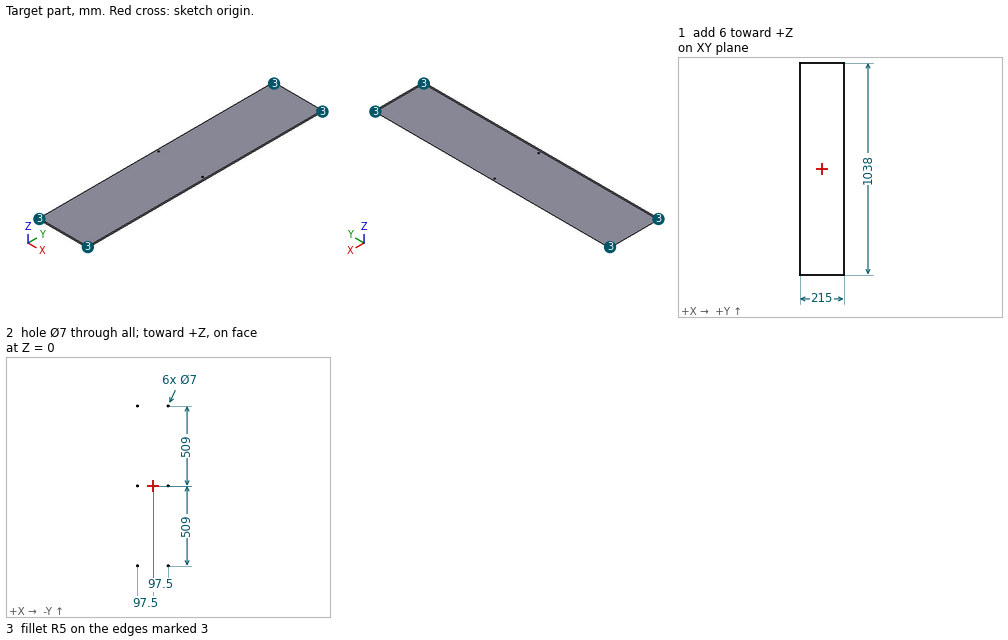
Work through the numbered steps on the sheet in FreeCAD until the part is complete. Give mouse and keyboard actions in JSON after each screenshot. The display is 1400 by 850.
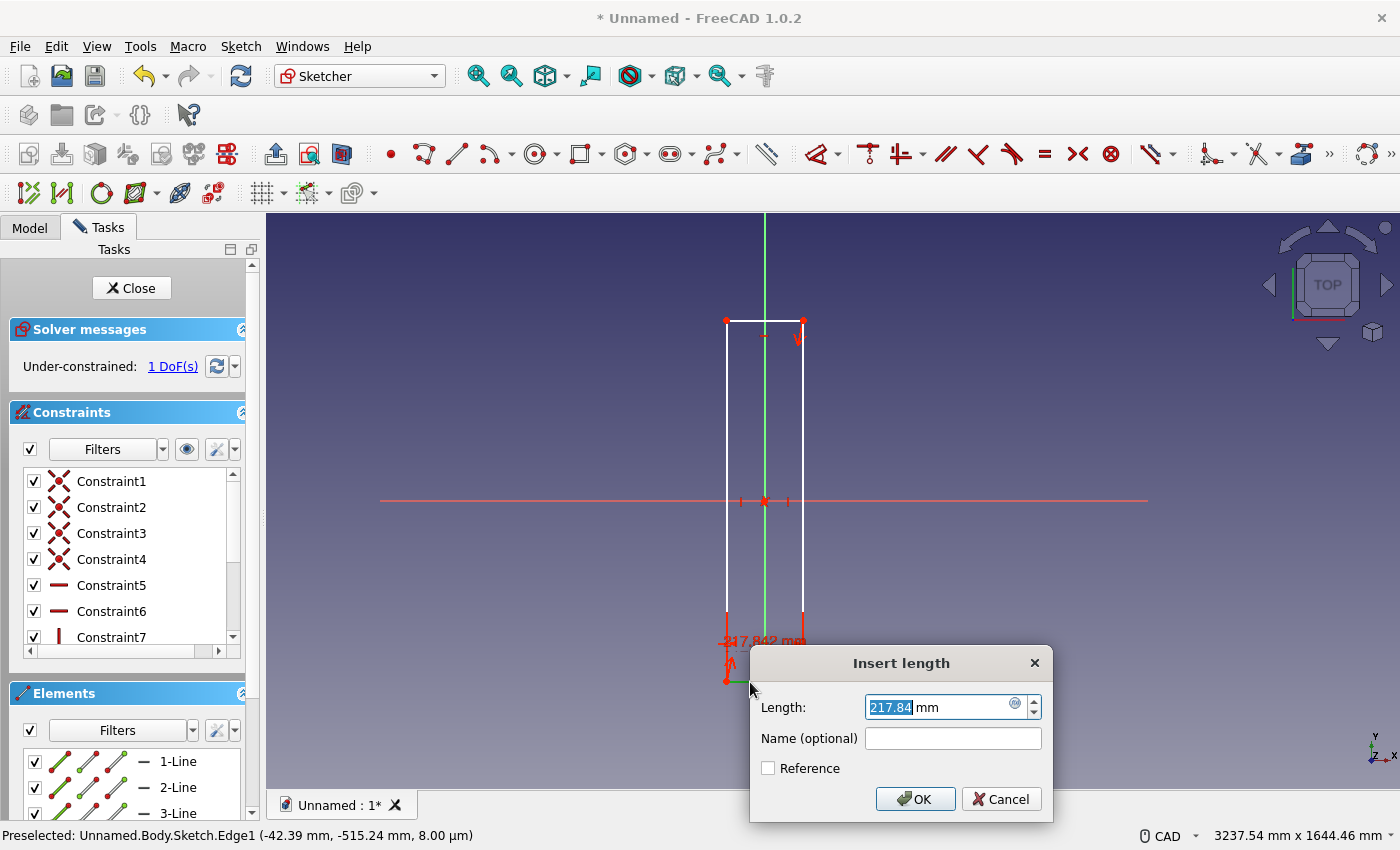
{"action": "type", "text": "215"}
{"action": "key", "text": "Return"}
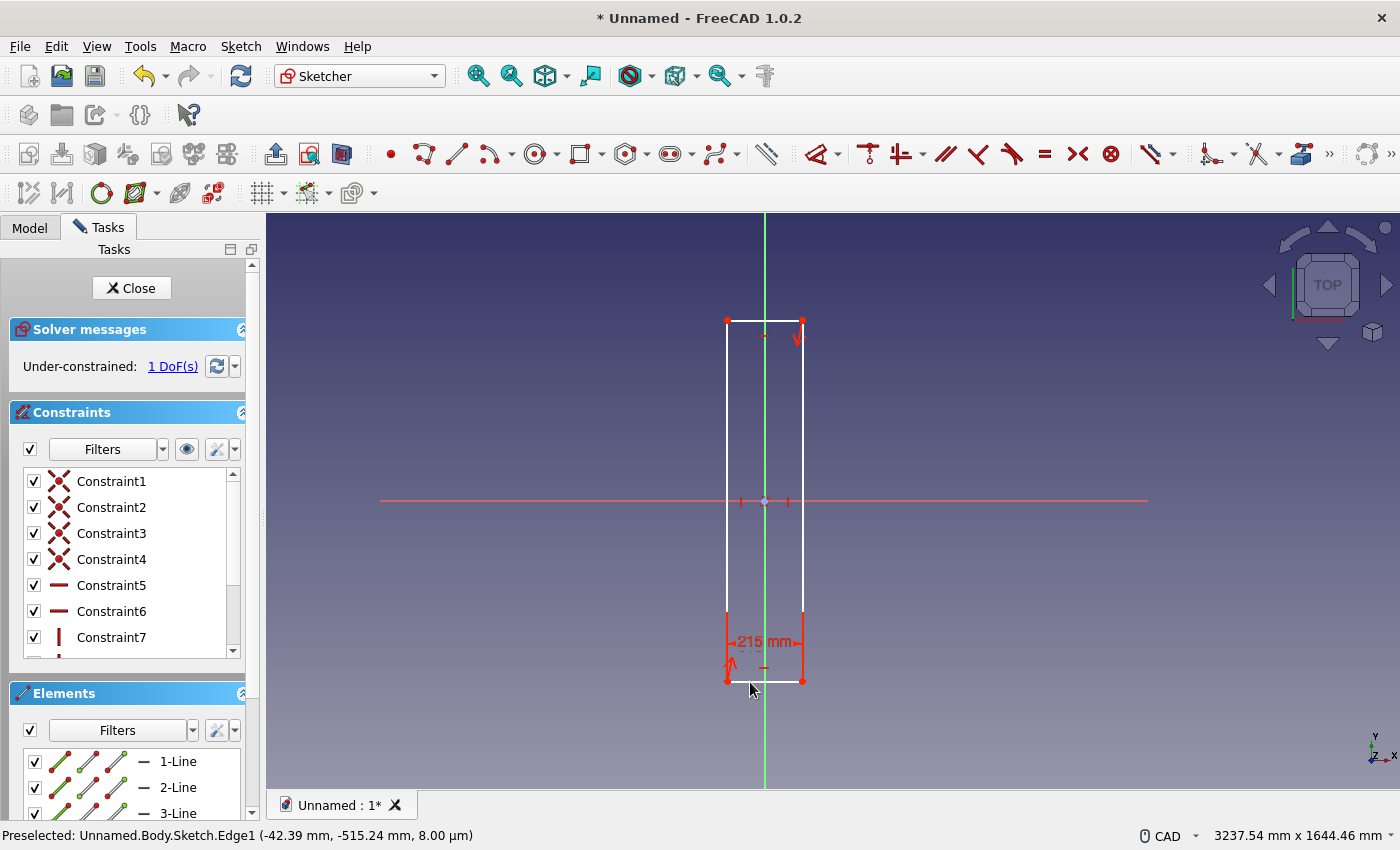
{"action": "left_click", "coordinate": [803, 574]}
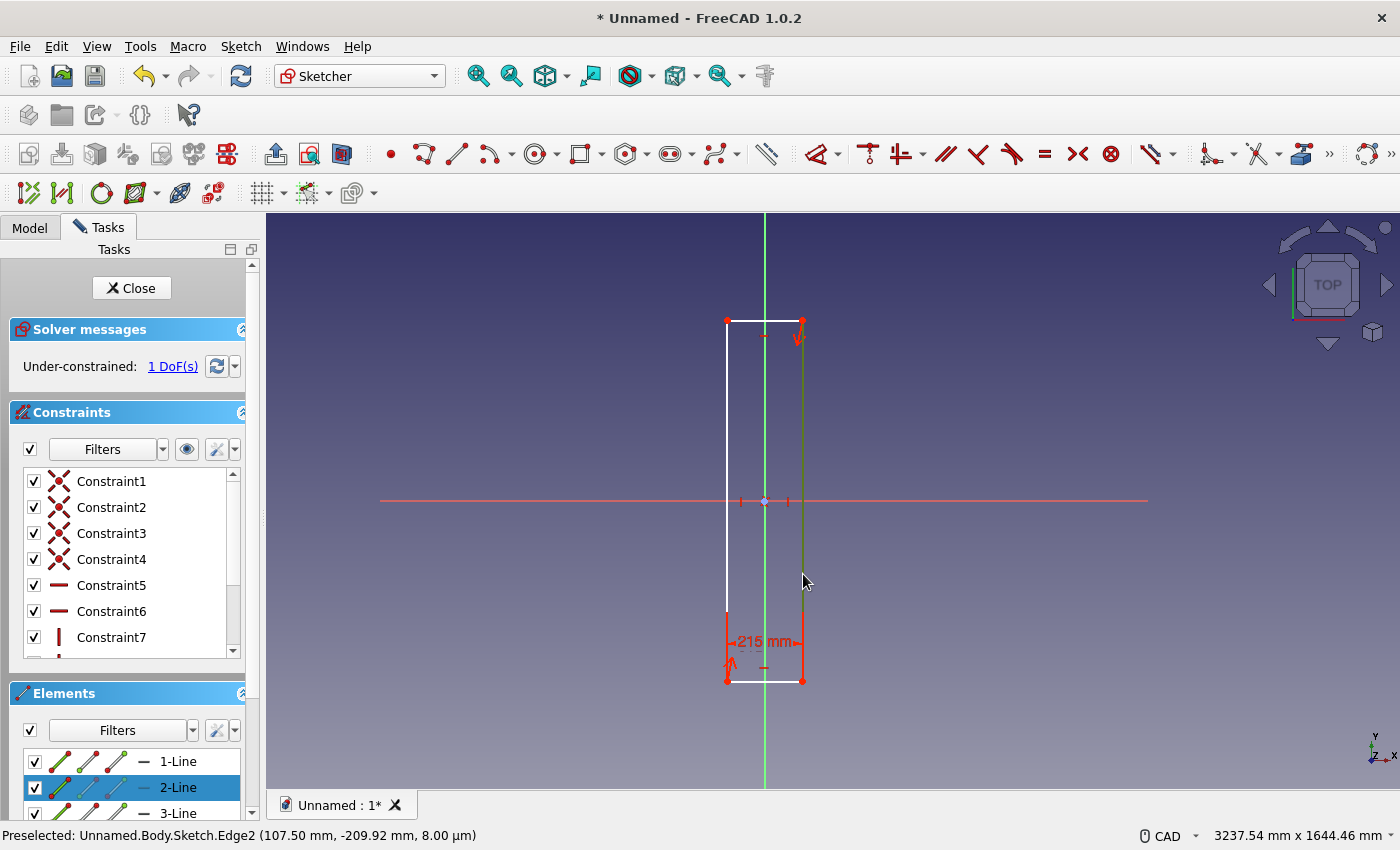
{"action": "key", "text": "i"}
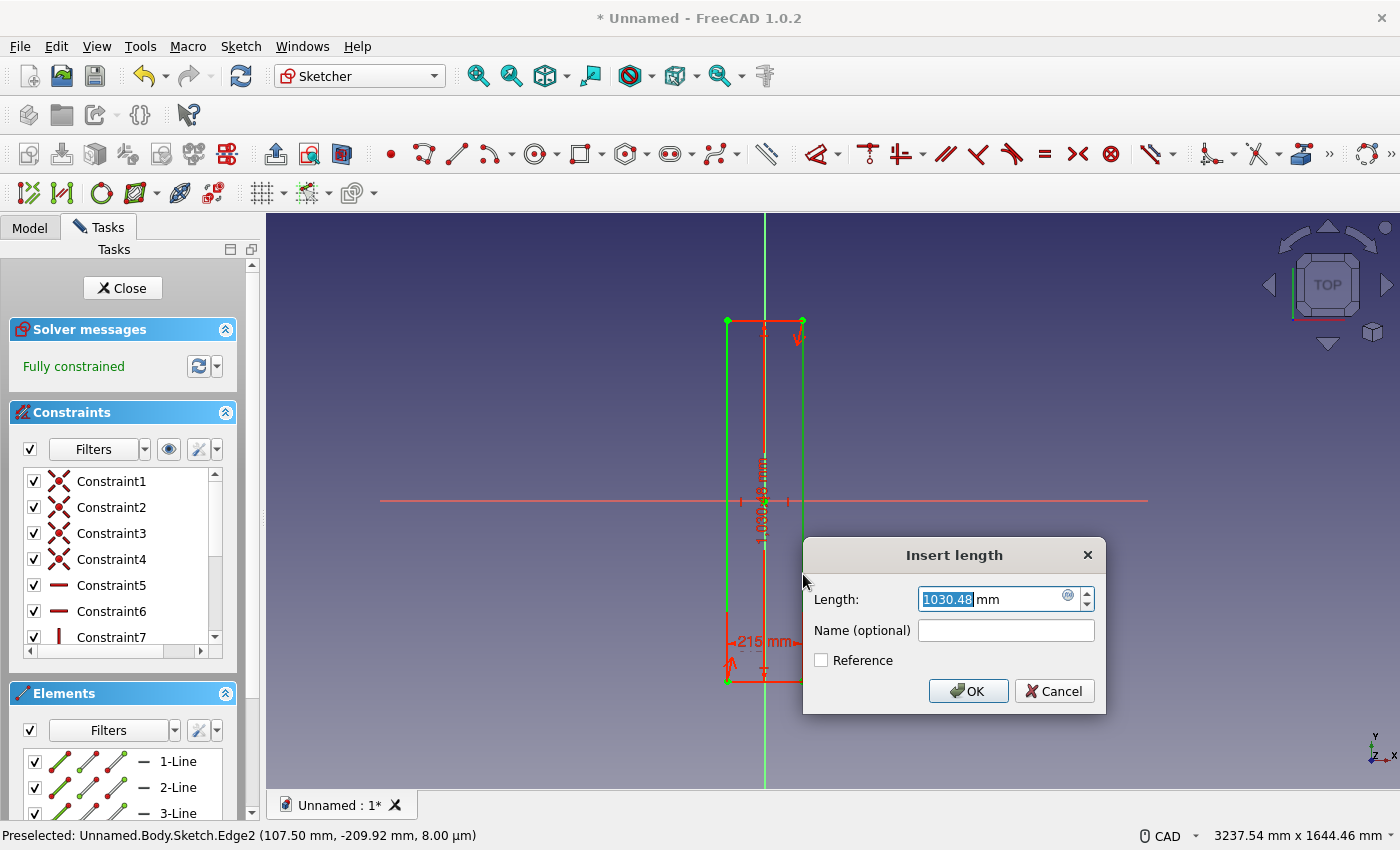
{"action": "type", "text": "1038"}
{"action": "key", "text": "Return"}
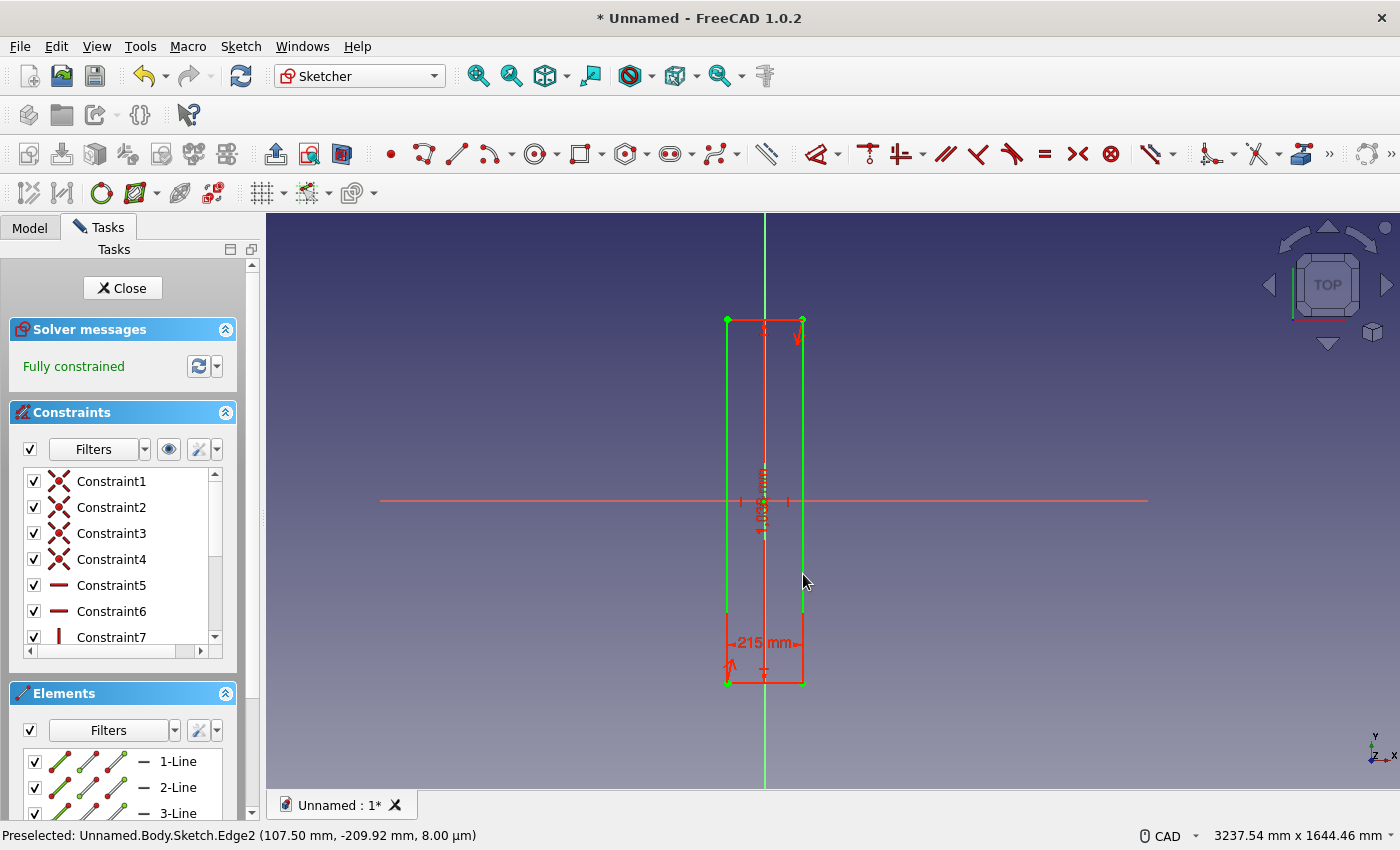
{"action": "left_click", "coordinate": [123, 288]}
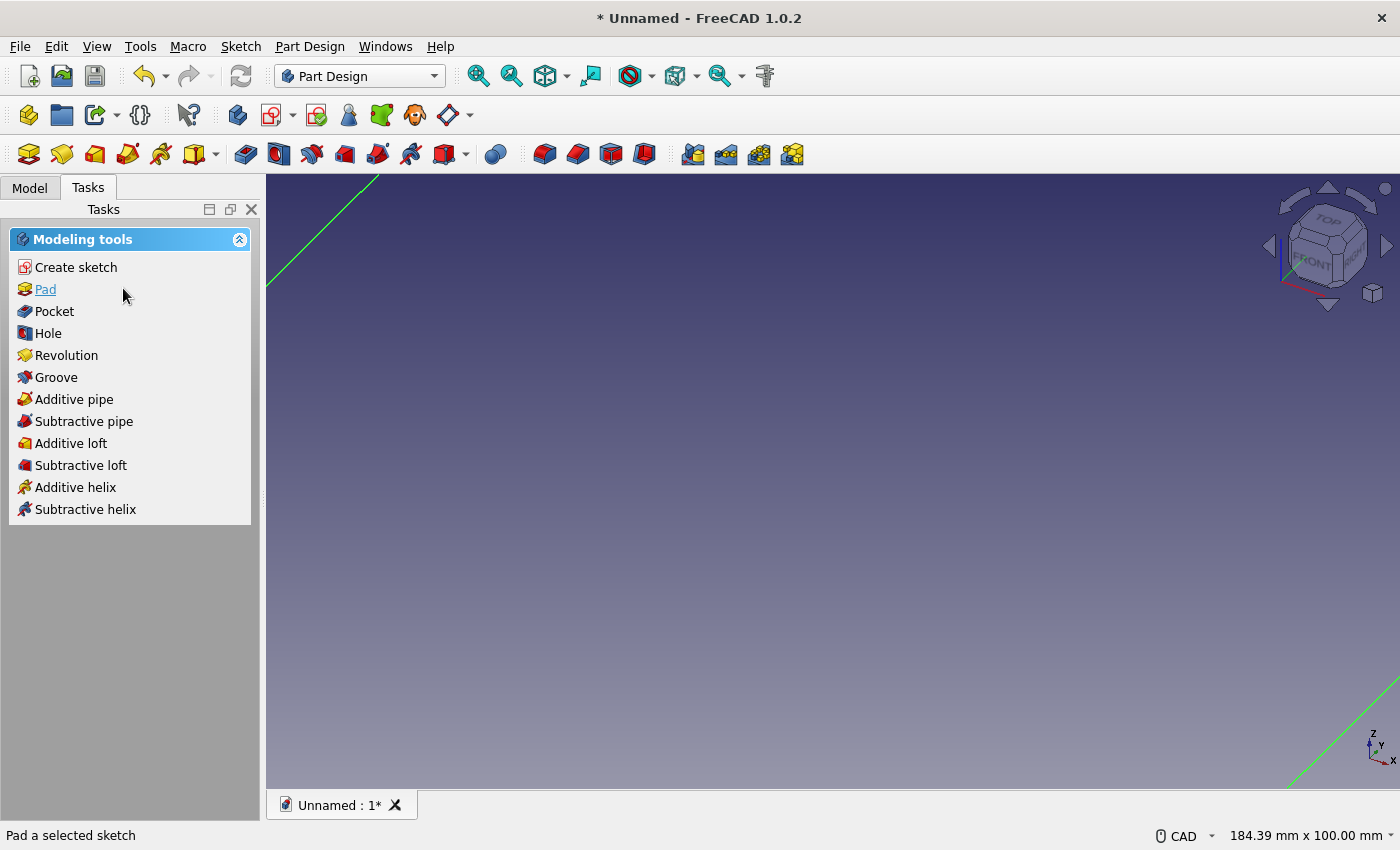
{"action": "left_click", "coordinate": [29, 154]}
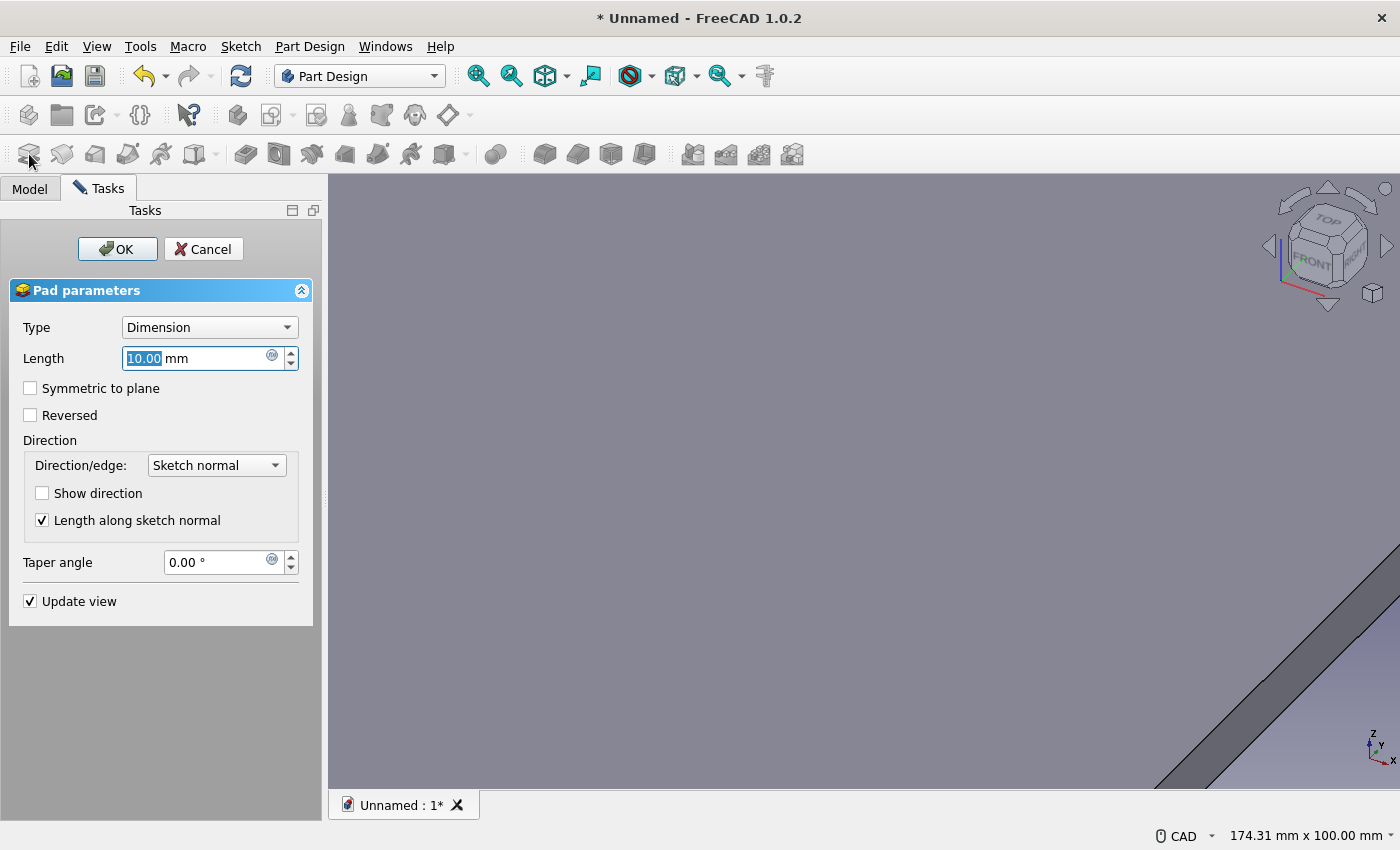
{"action": "type", "text": "6"}
{"action": "key", "text": "Tab"}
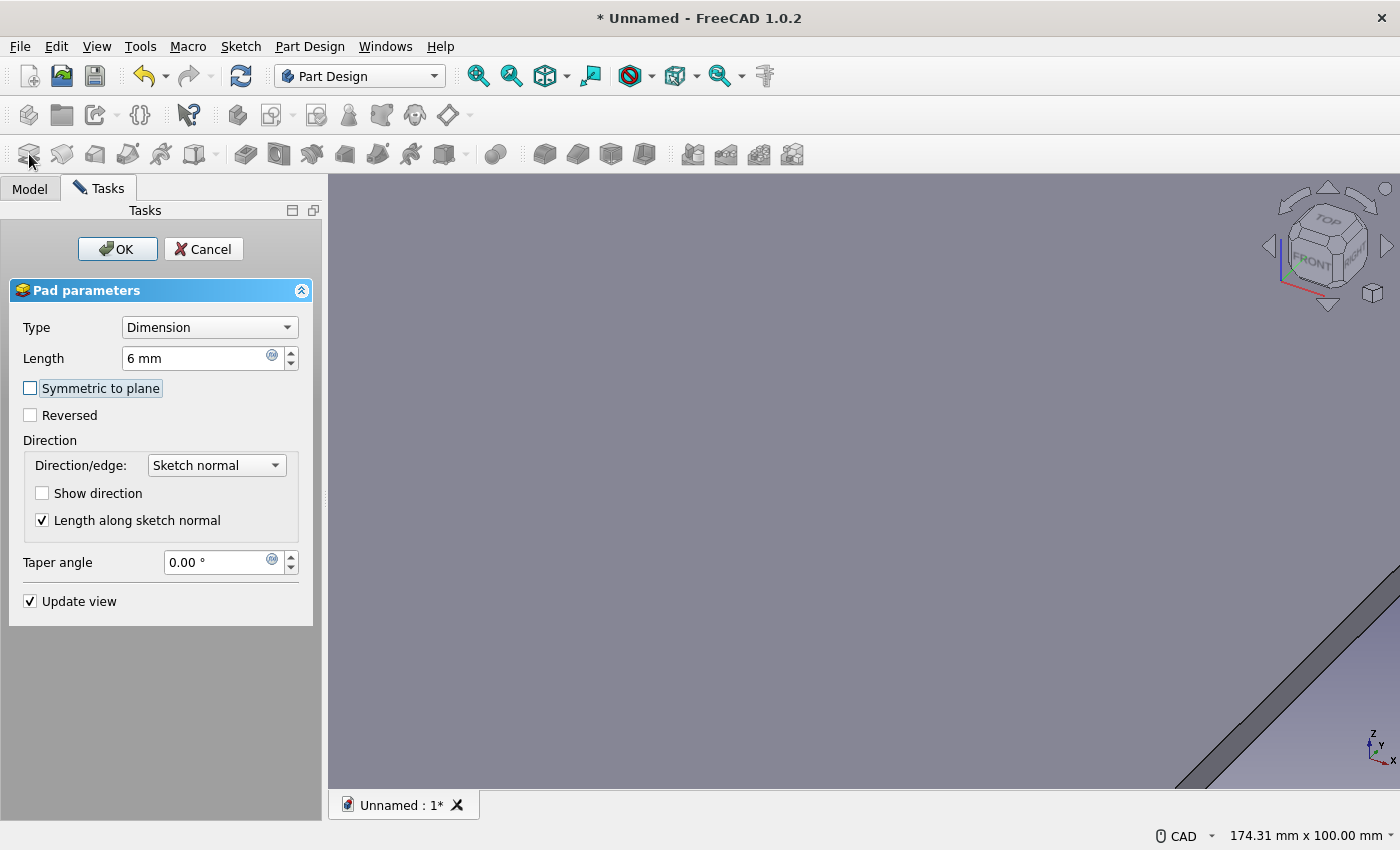
{"action": "left_click", "coordinate": [118, 249]}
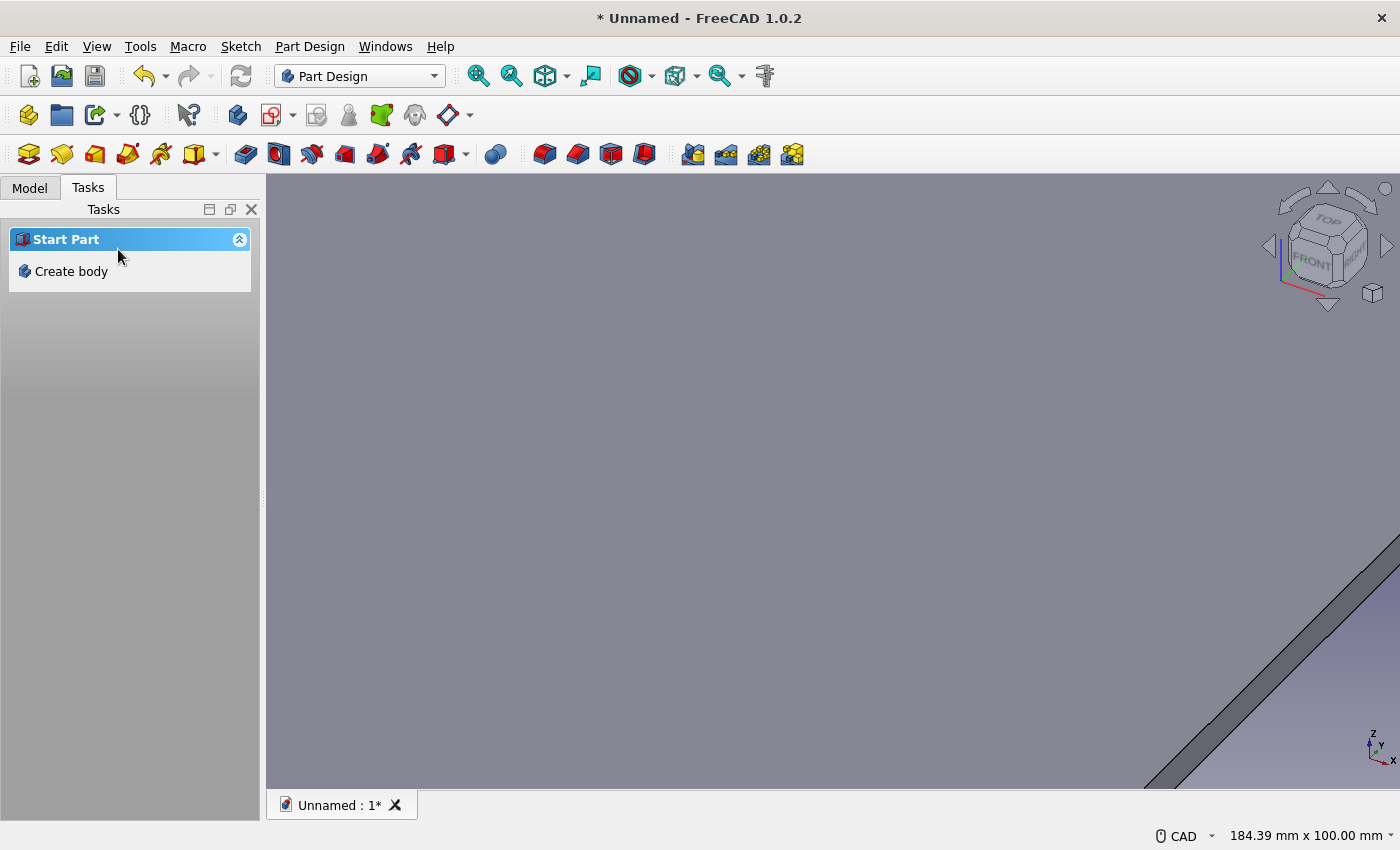
{"action": "left_click", "coordinate": [479, 76]}